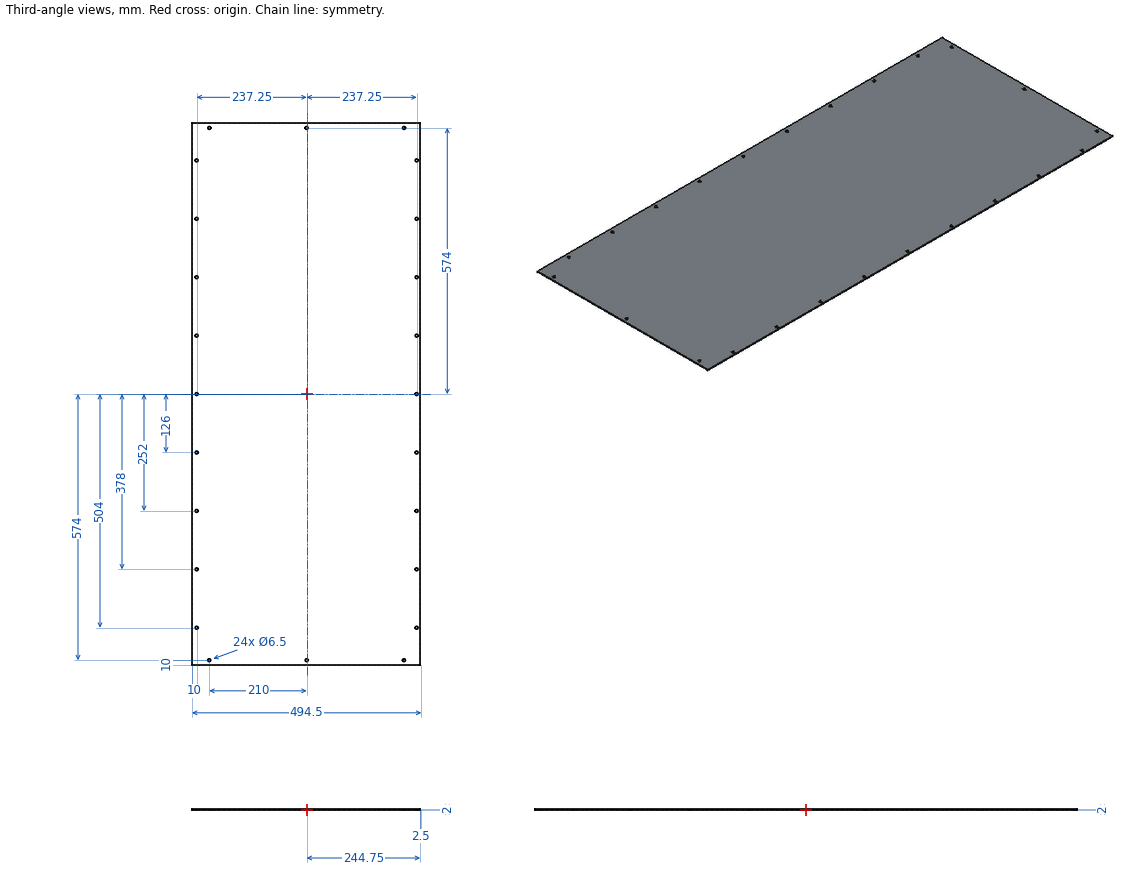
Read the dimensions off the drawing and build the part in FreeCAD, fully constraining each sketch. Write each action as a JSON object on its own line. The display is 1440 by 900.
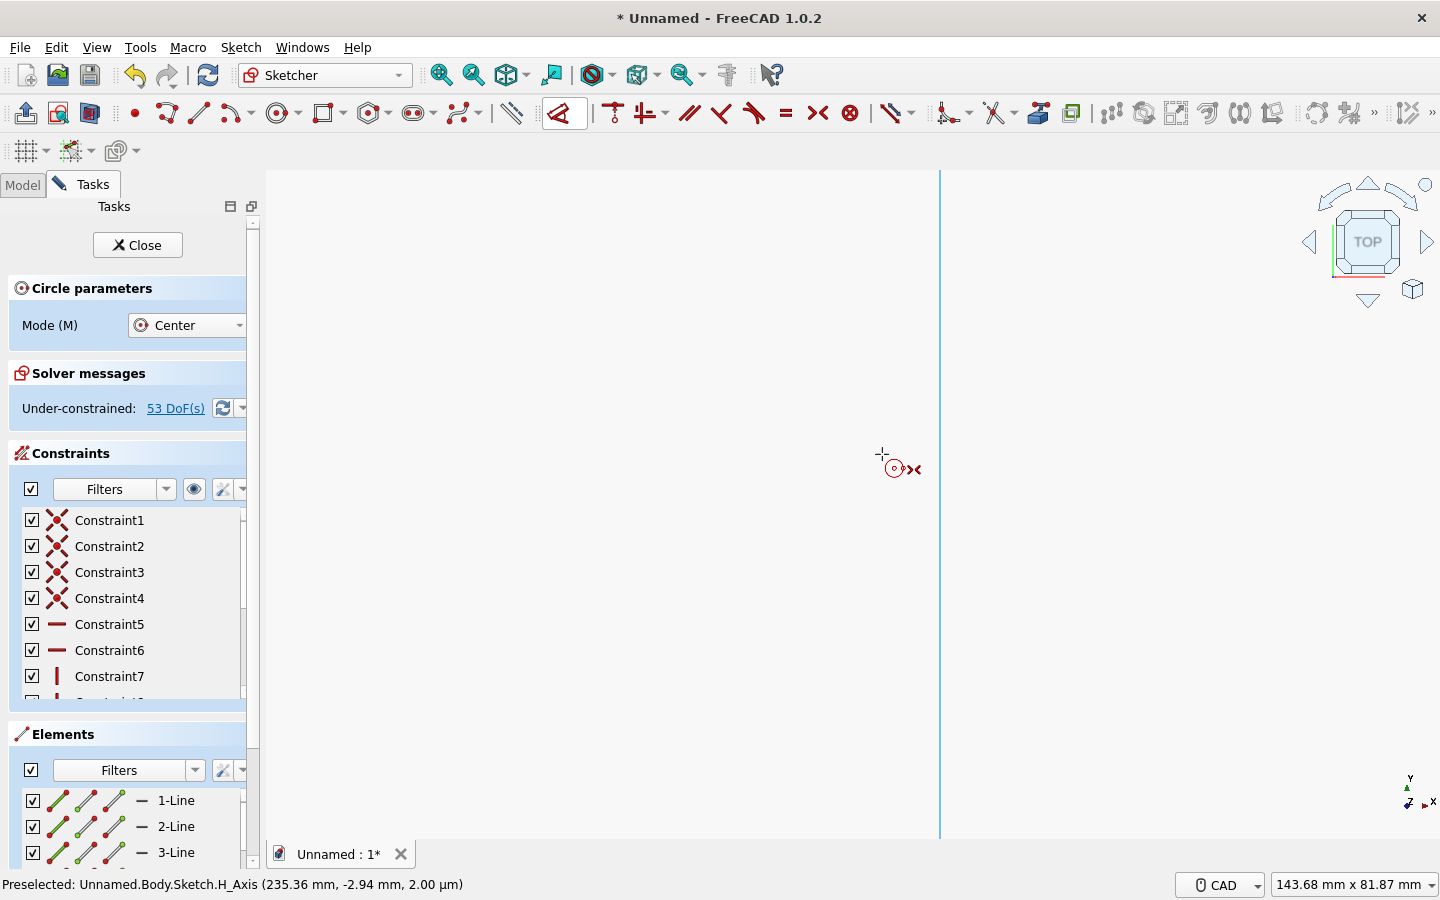
{"action": "scroll", "coordinate": [882, 454], "scroll_direction": "down", "scroll_amount": 15}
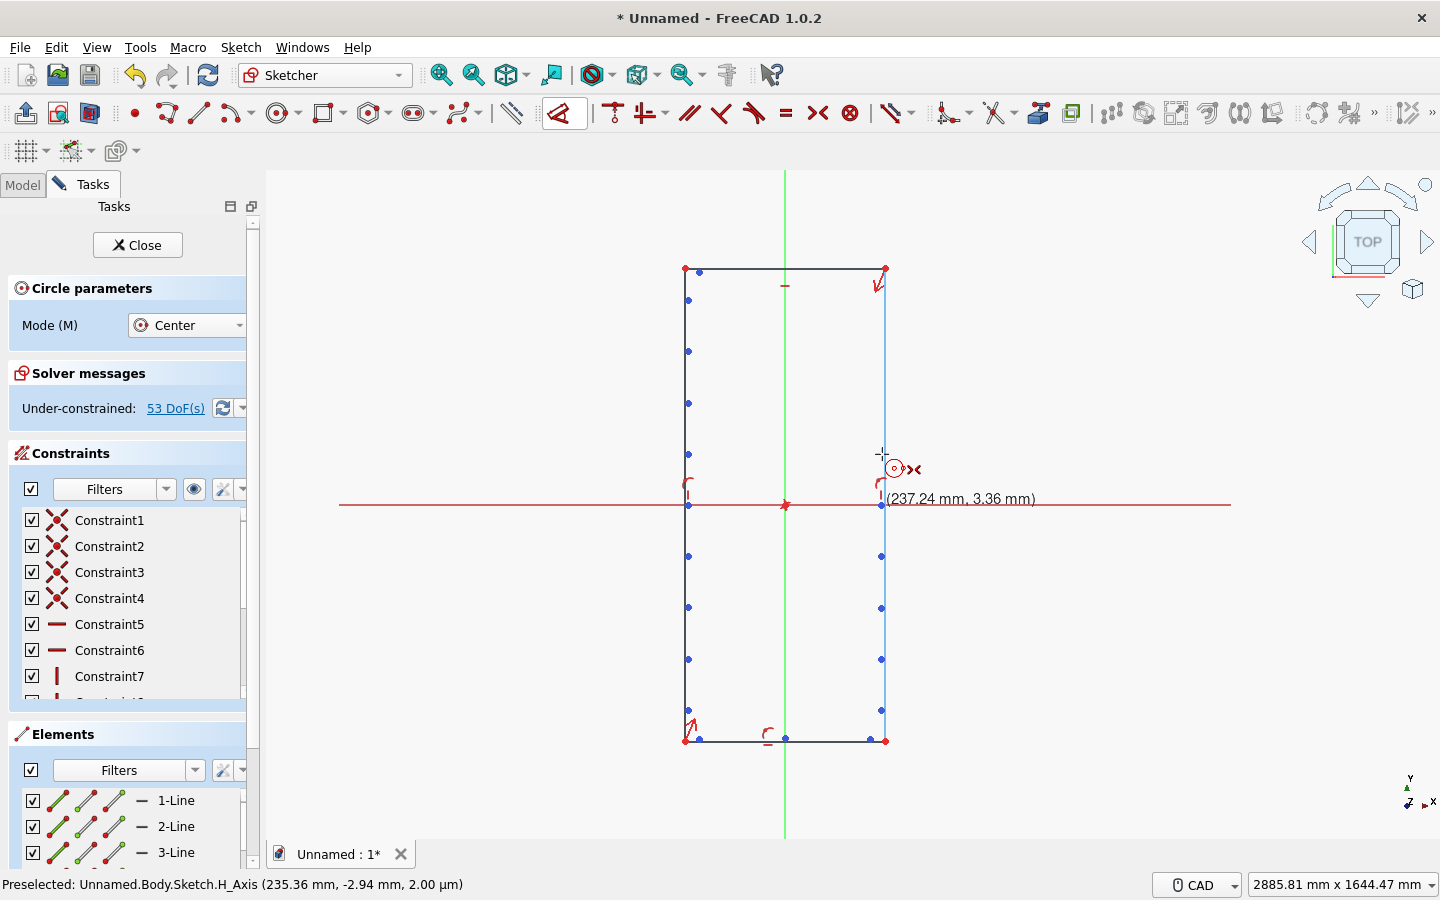
{"action": "scroll", "coordinate": [882, 454], "scroll_direction": "up", "scroll_amount": 7}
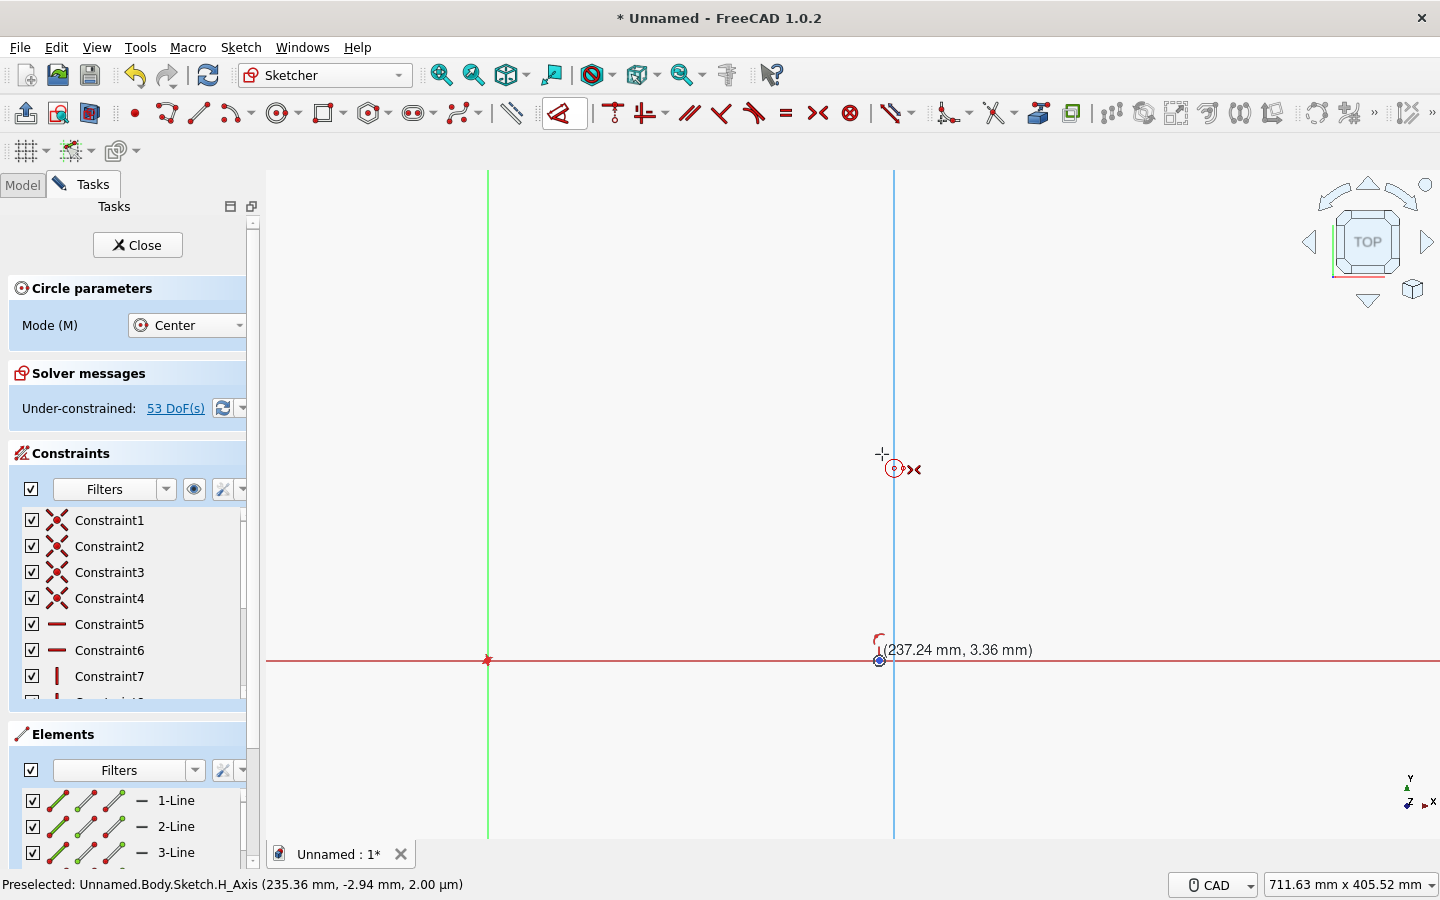
{"action": "left_click", "coordinate": [879, 453]}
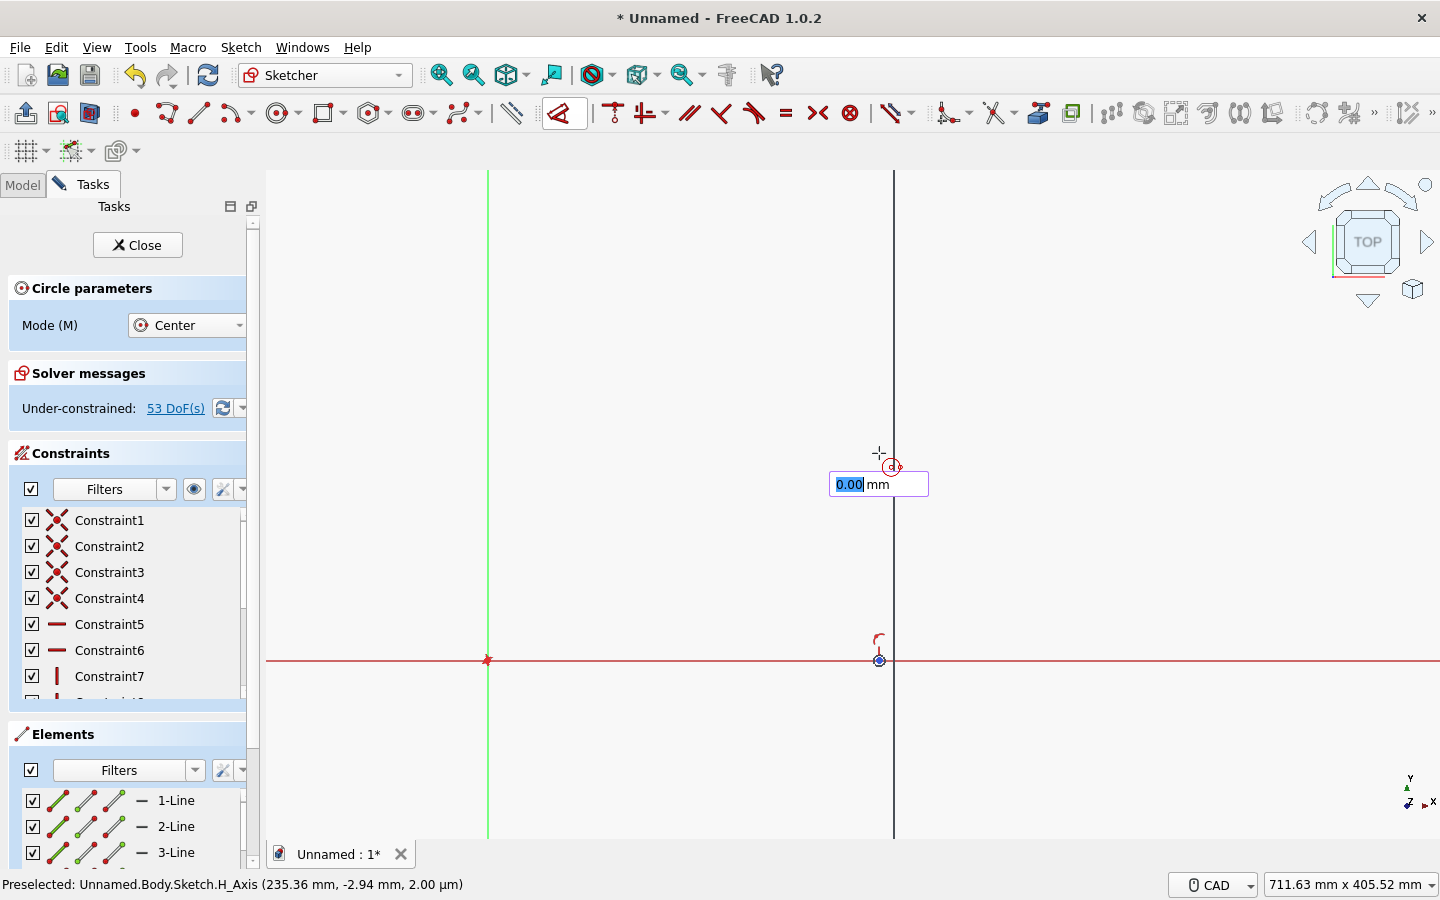
{"action": "scroll", "coordinate": [876, 449], "scroll_direction": "up", "scroll_amount": 6}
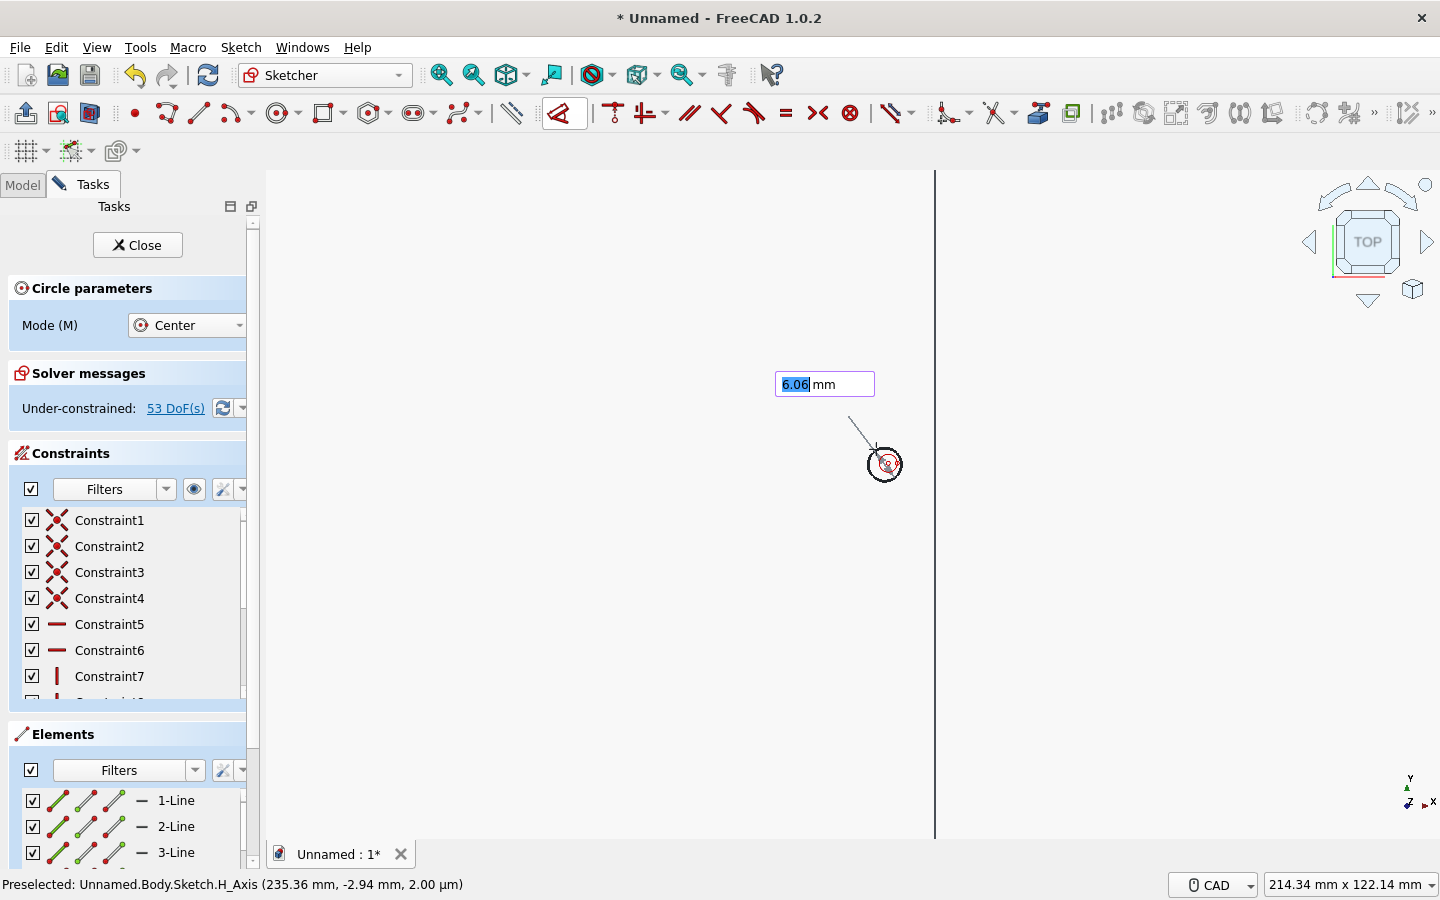
{"action": "left_click", "coordinate": [873, 449]}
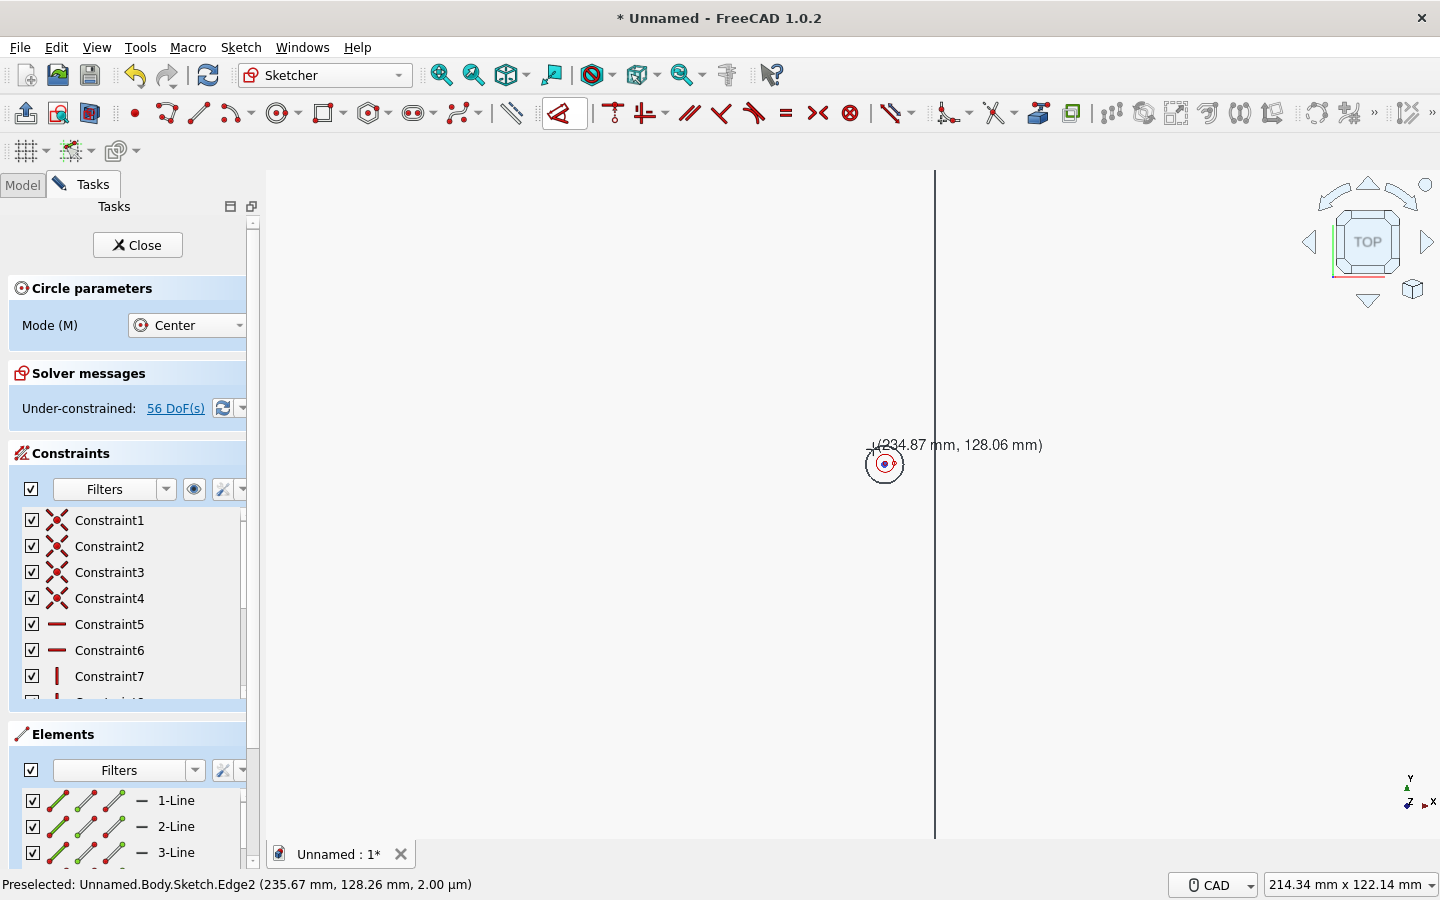
{"action": "scroll", "coordinate": [881, 453], "scroll_direction": "down", "scroll_amount": 13}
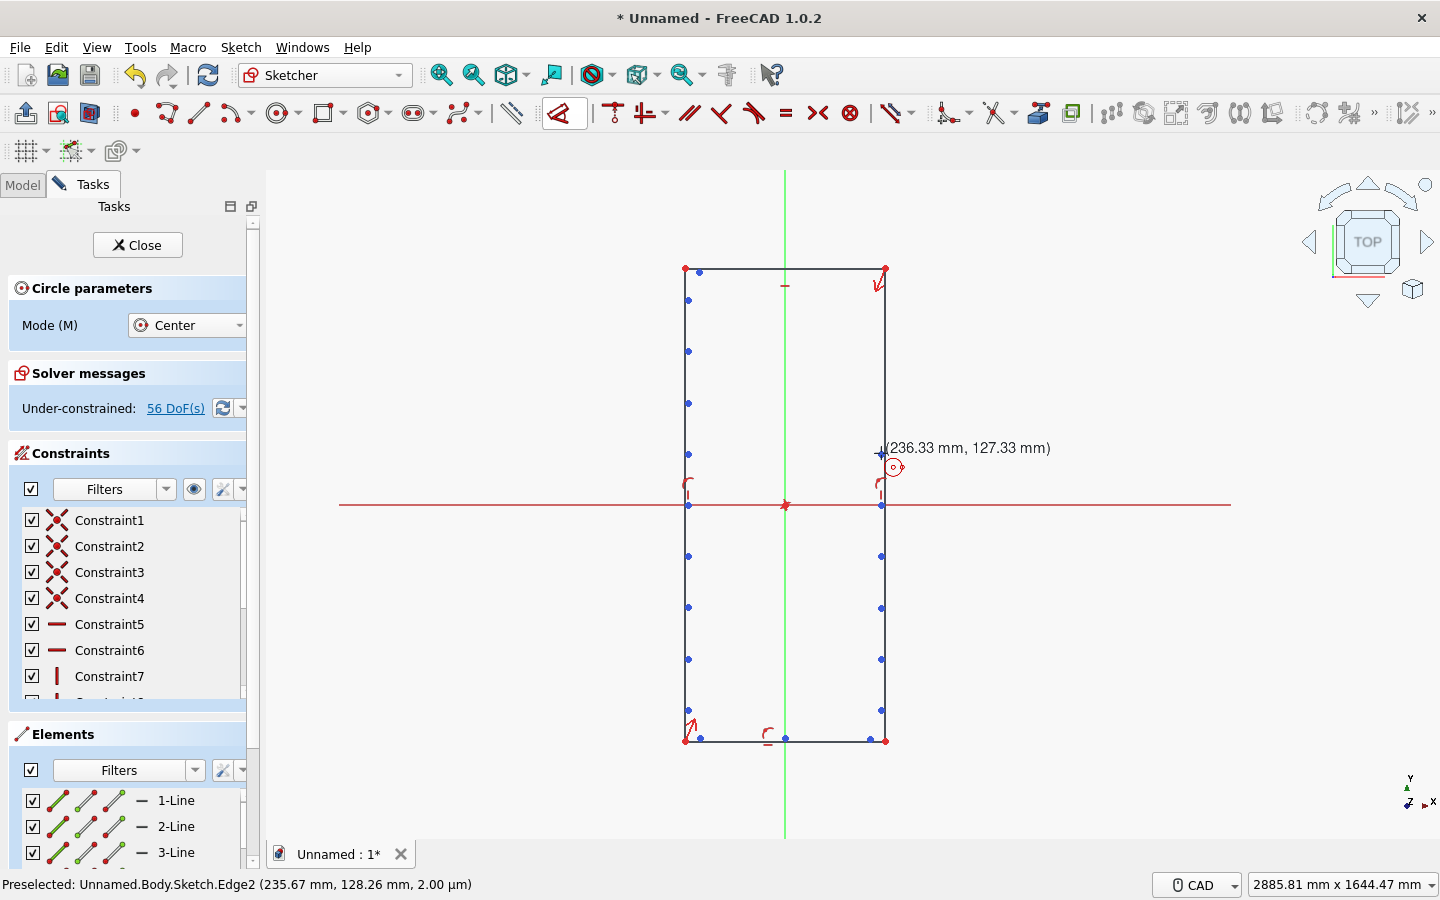
{"action": "scroll", "coordinate": [882, 403], "scroll_direction": "up", "scroll_amount": 15}